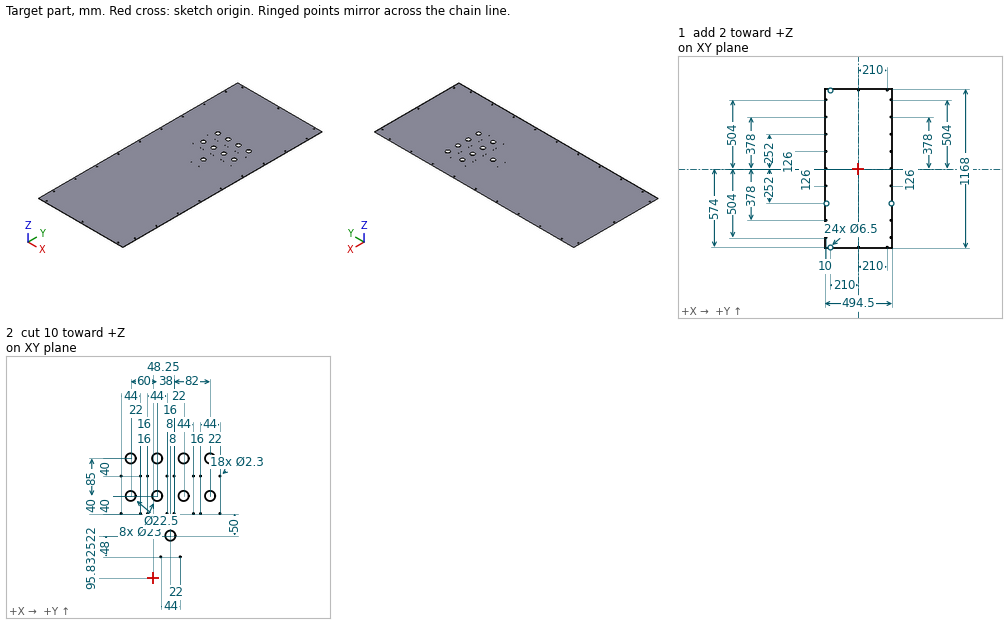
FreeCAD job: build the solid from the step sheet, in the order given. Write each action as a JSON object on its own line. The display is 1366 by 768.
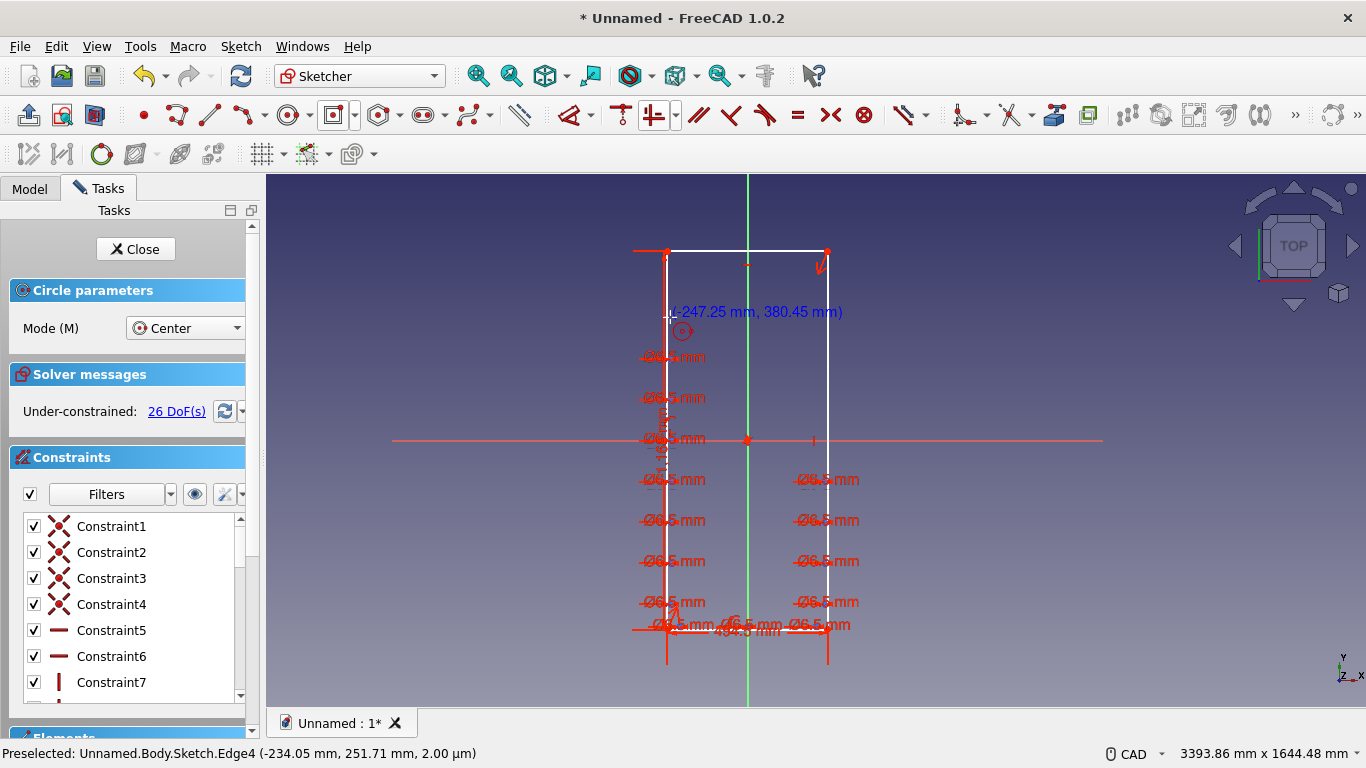
{"action": "scroll", "coordinate": [671, 318], "scroll_direction": "up", "scroll_amount": 8}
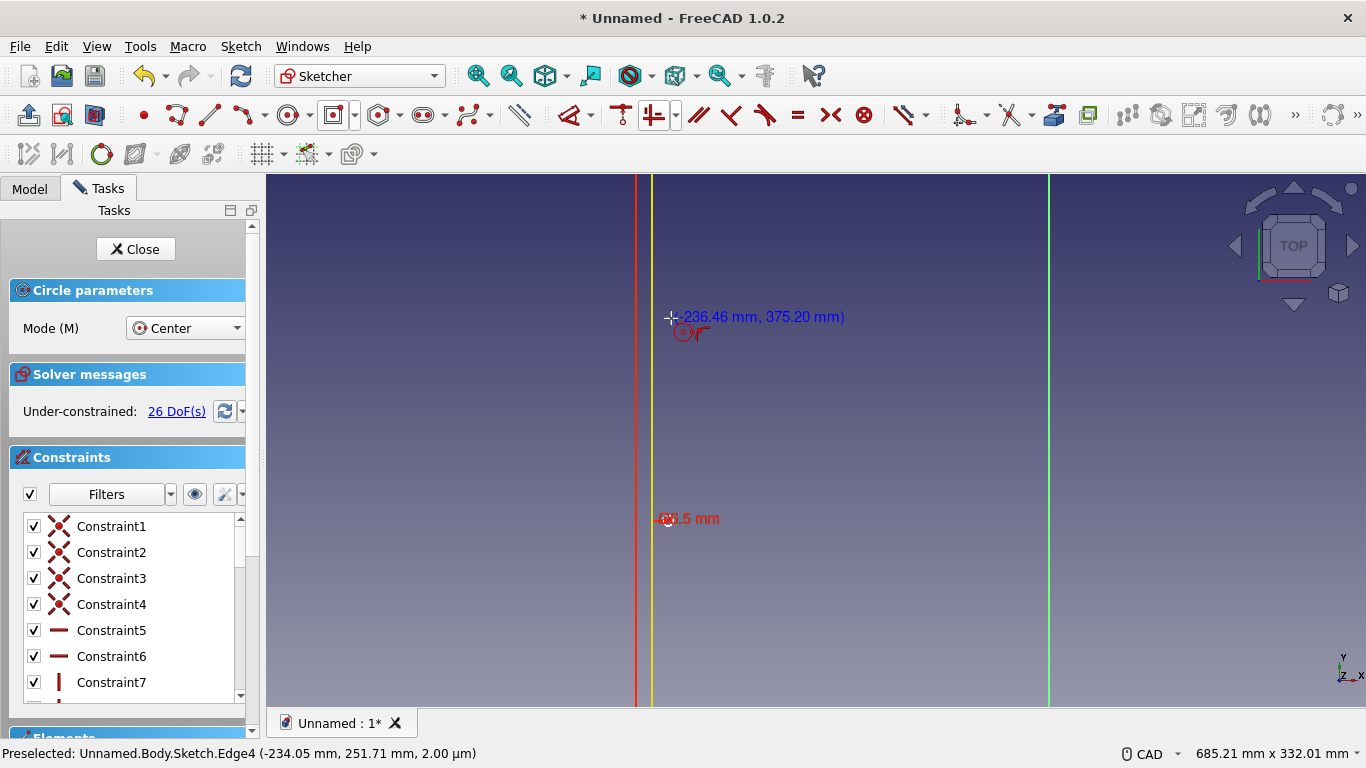
{"action": "left_click", "coordinate": [668, 317]}
{"action": "mouse_move", "coordinate": [672, 314]}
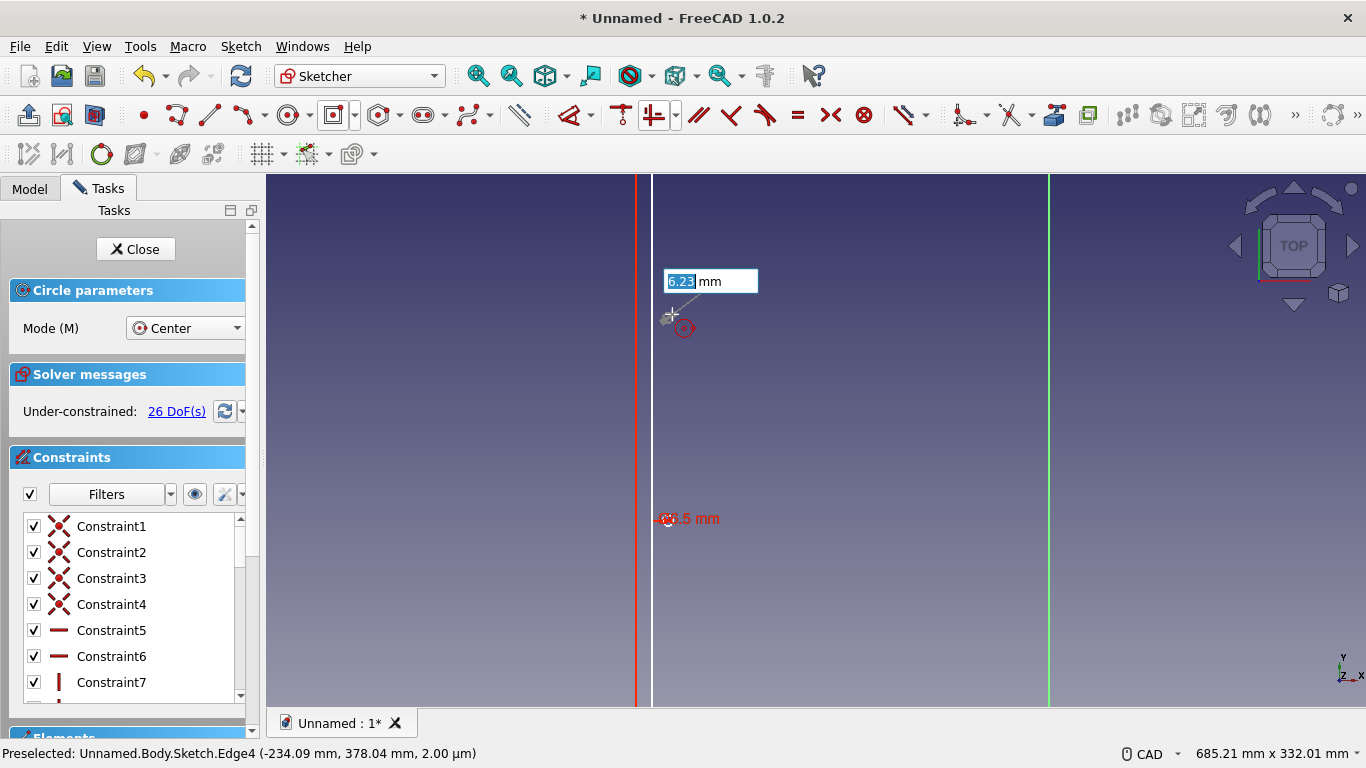
{"action": "type", "text": "6.5"}
{"action": "key", "text": "Return"}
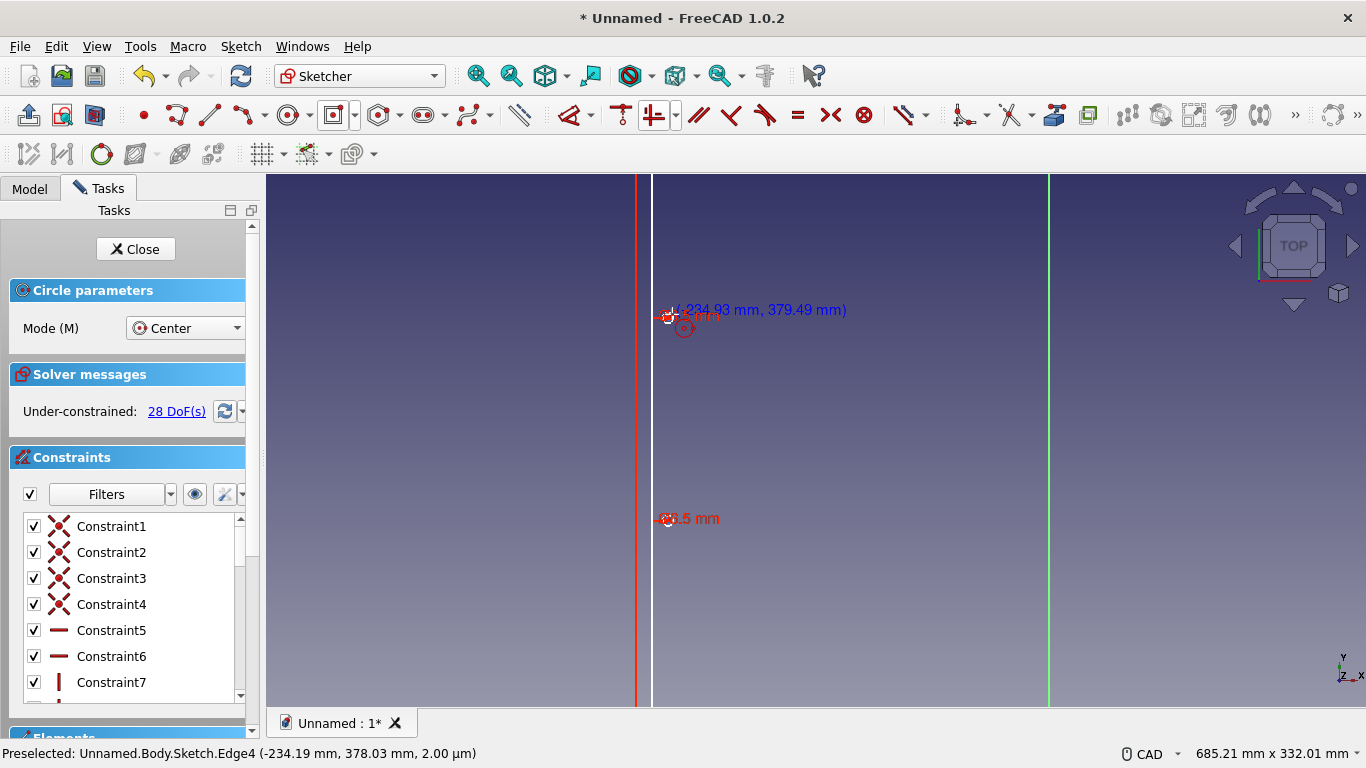
{"action": "scroll", "coordinate": [688, 345], "scroll_direction": "down", "scroll_amount": 9}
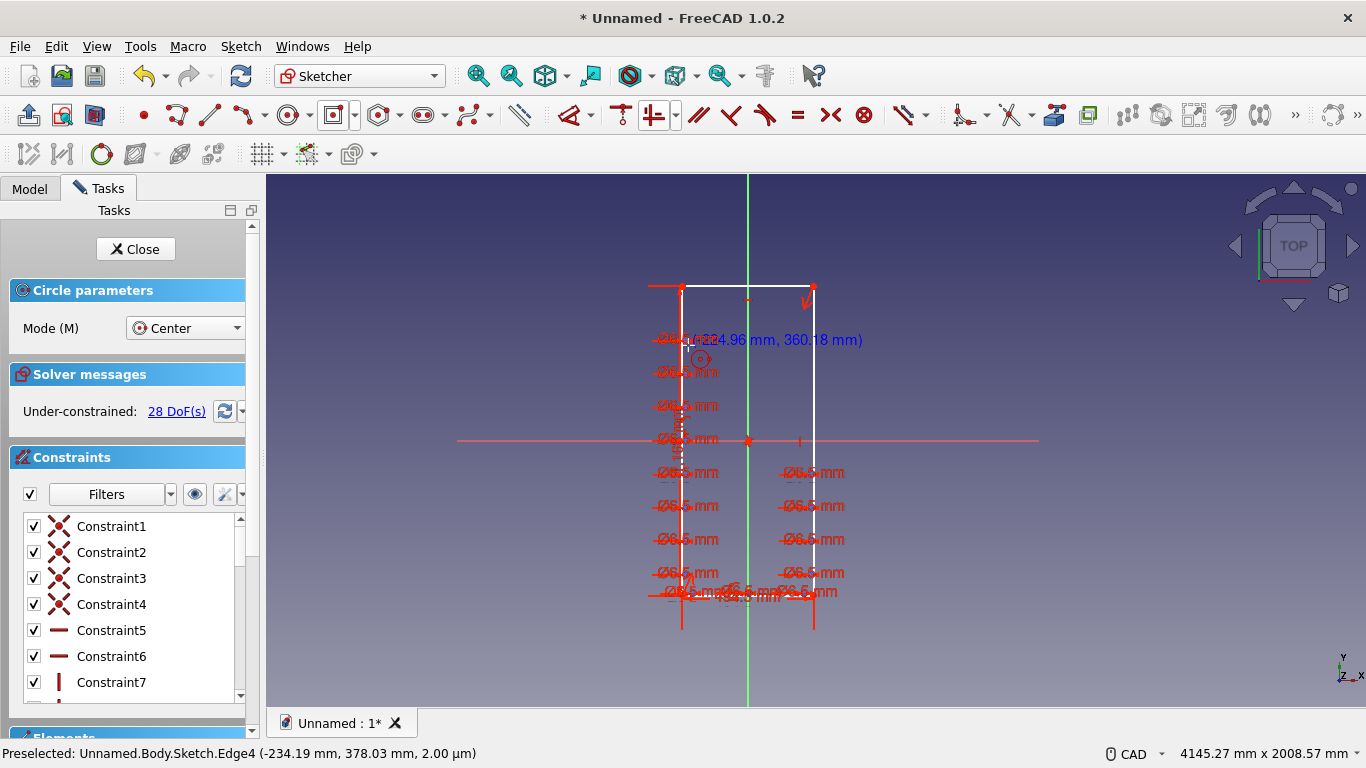
{"action": "scroll", "coordinate": [685, 307], "scroll_direction": "up", "scroll_amount": 17}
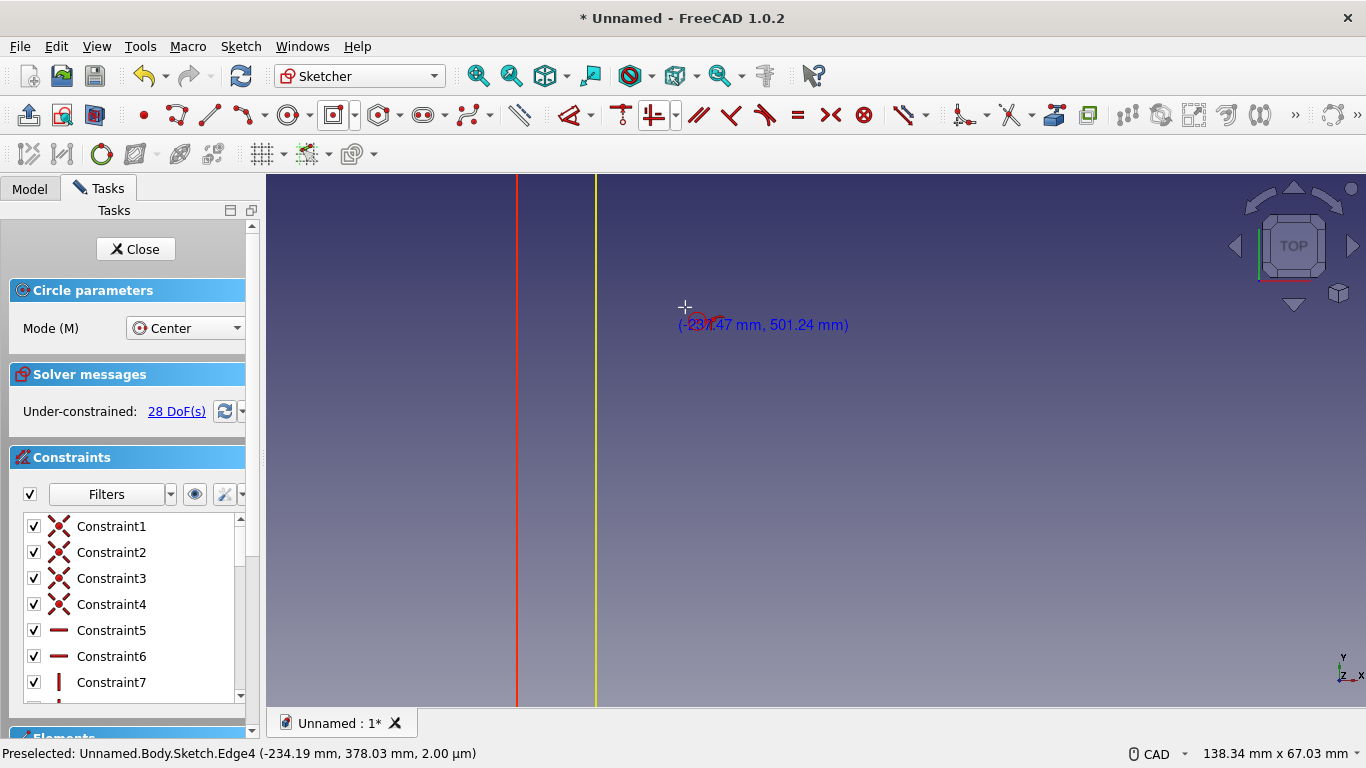
{"action": "scroll", "coordinate": [670, 276], "scroll_direction": "down", "scroll_amount": 16}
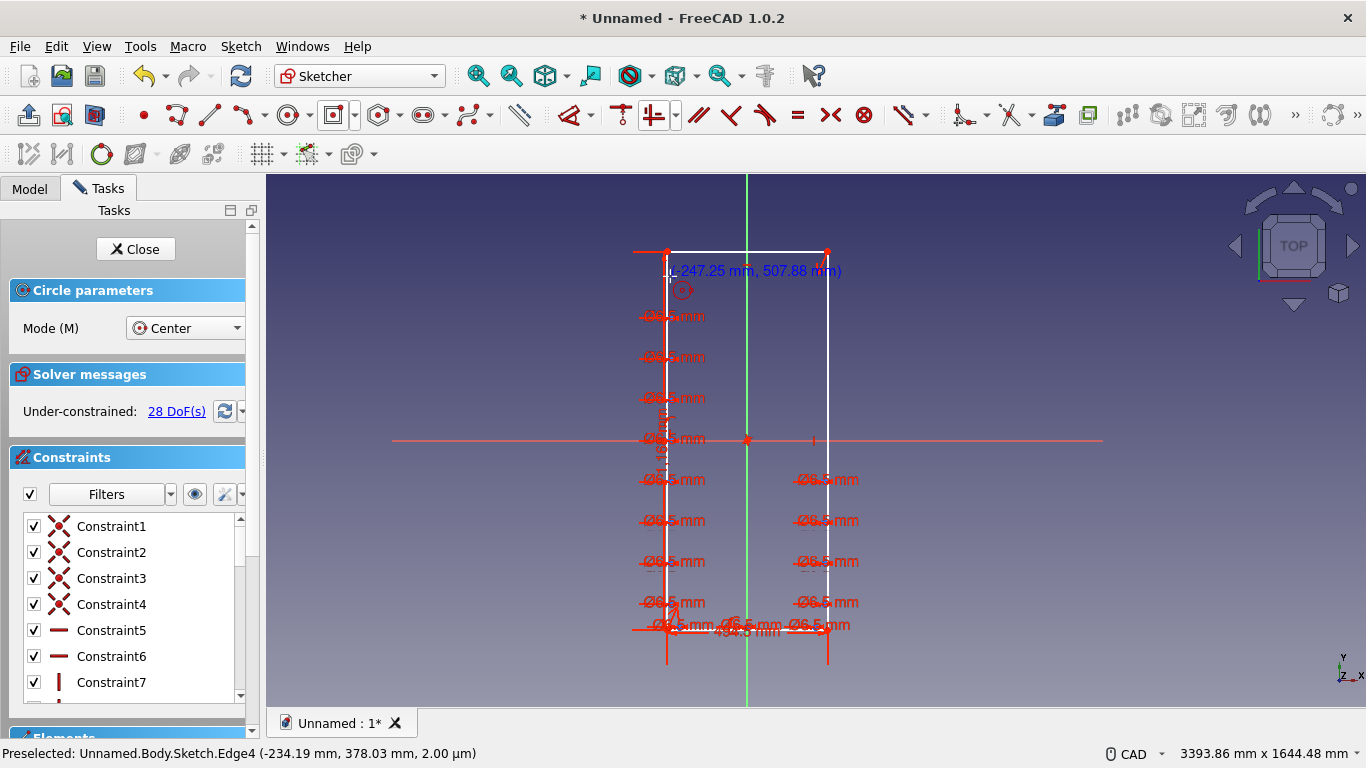
{"action": "scroll", "coordinate": [671, 277], "scroll_direction": "up", "scroll_amount": 8}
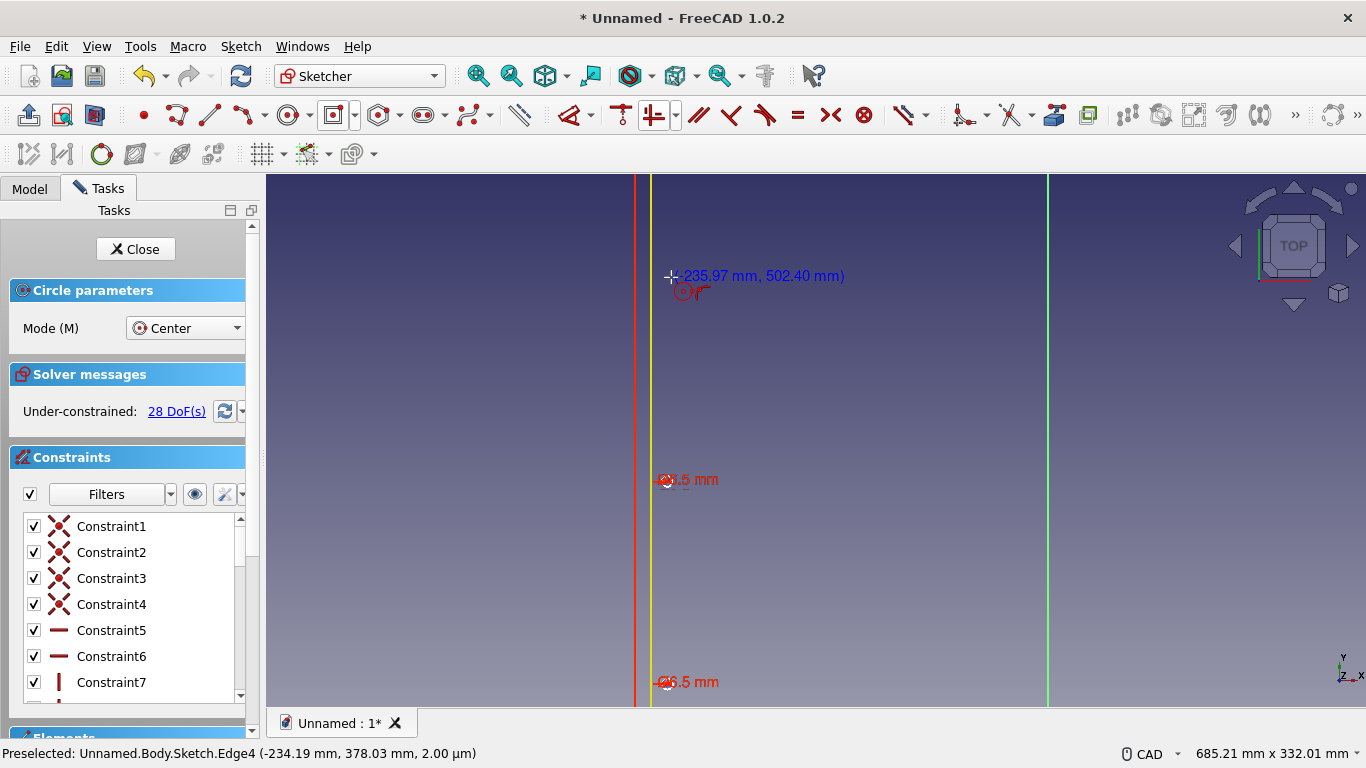
{"action": "left_click", "coordinate": [667, 279]}
{"action": "mouse_move", "coordinate": [671, 275]}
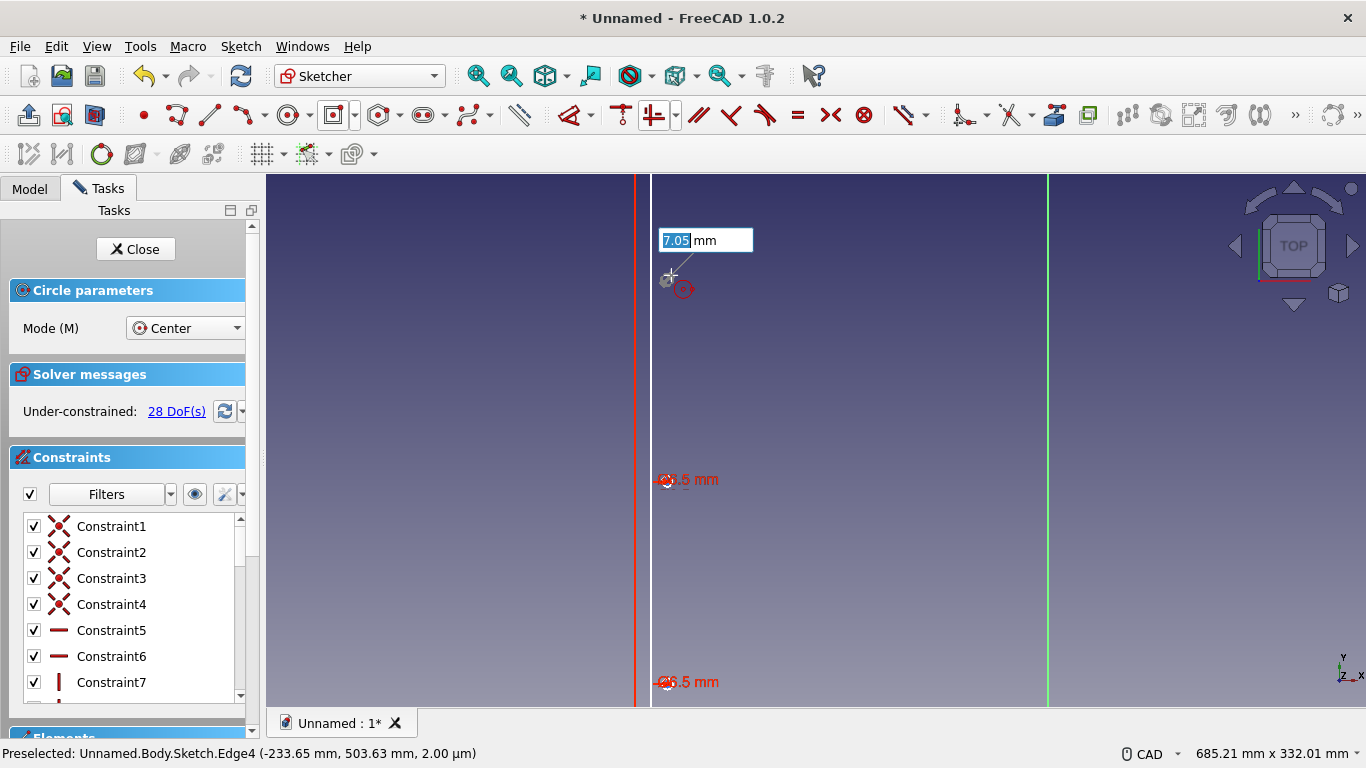
{"action": "type", "text": "6.5"}
{"action": "key", "text": "Return"}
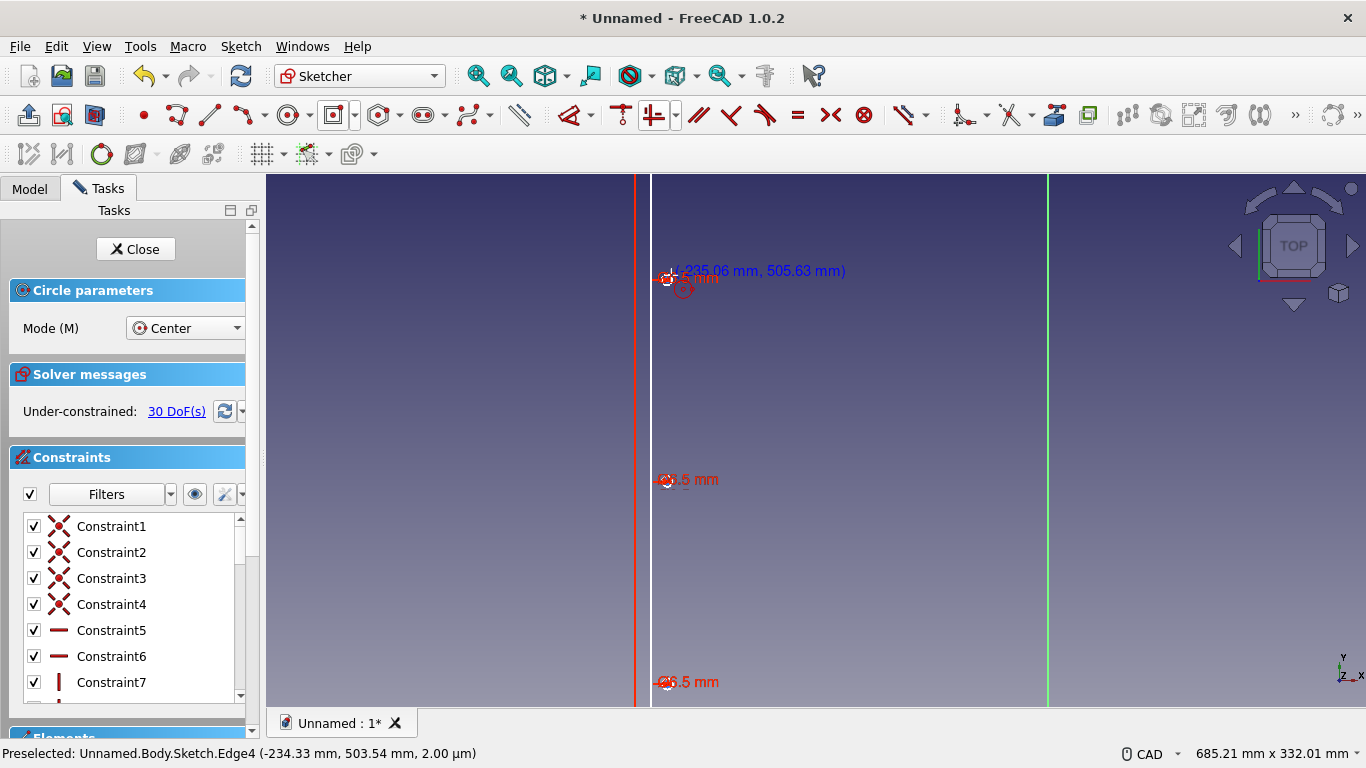
{"action": "scroll", "coordinate": [688, 312], "scroll_direction": "down", "scroll_amount": 9}